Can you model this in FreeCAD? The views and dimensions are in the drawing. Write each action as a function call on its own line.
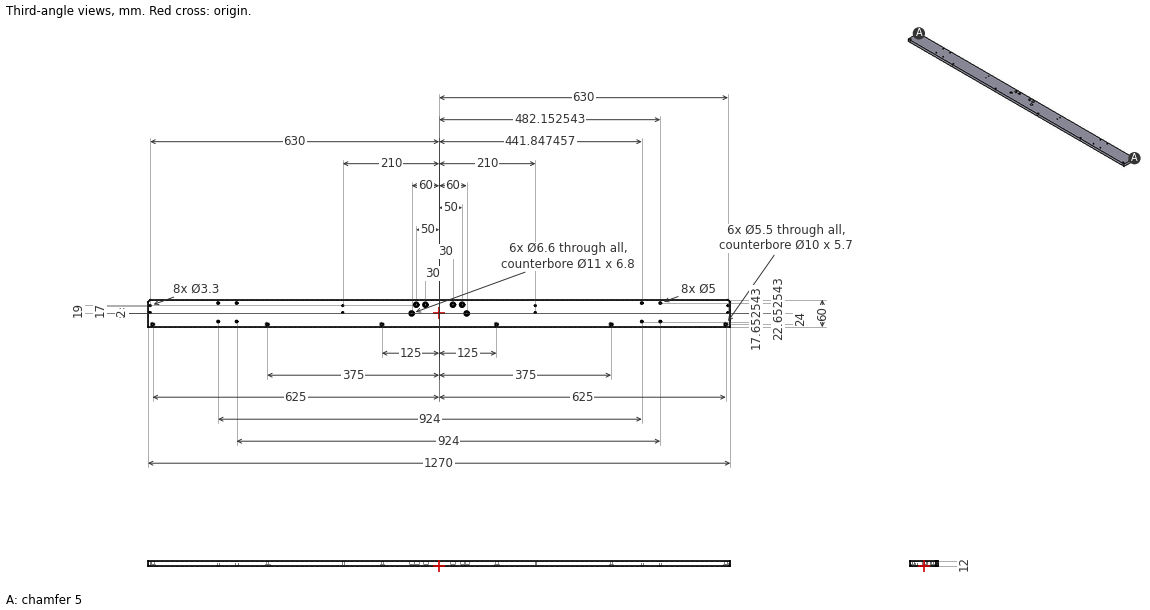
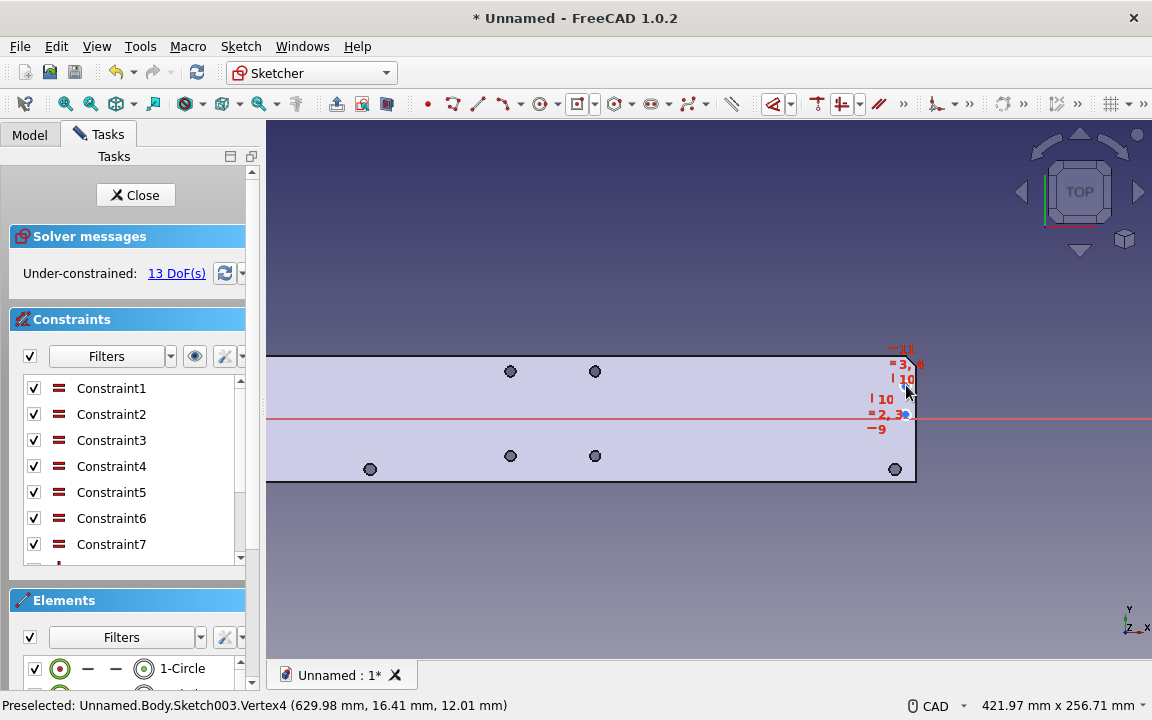
scroll(908, 387, down, 8)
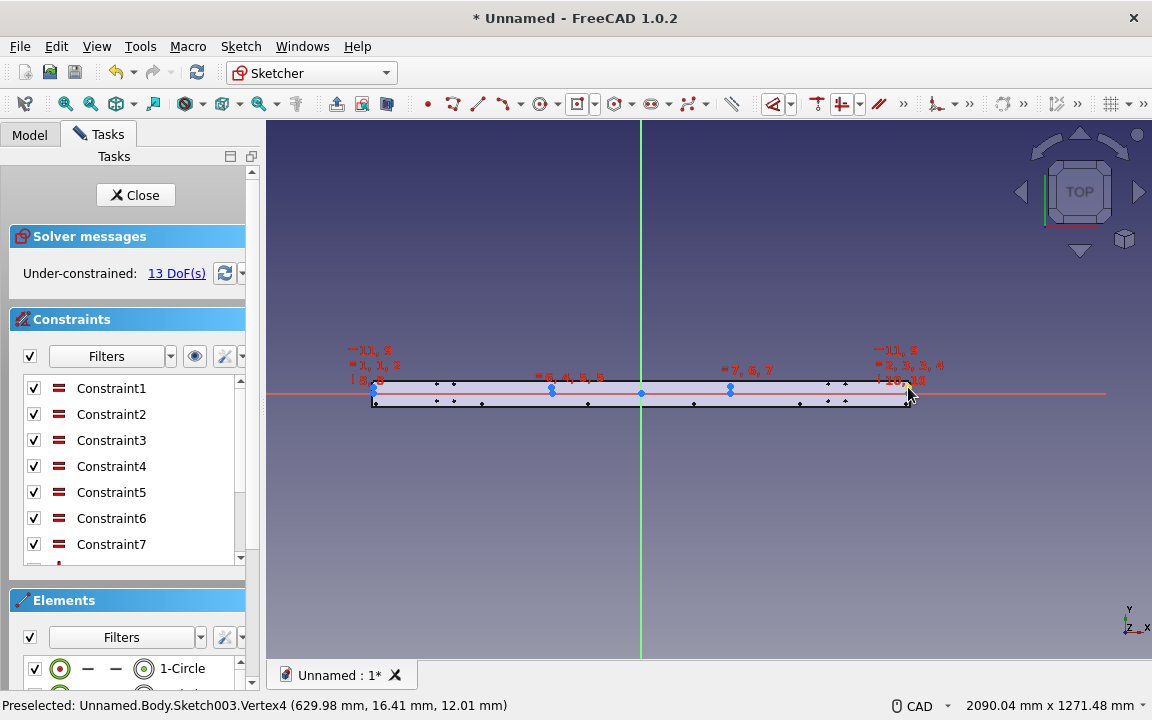
scroll(374, 387, up, 4)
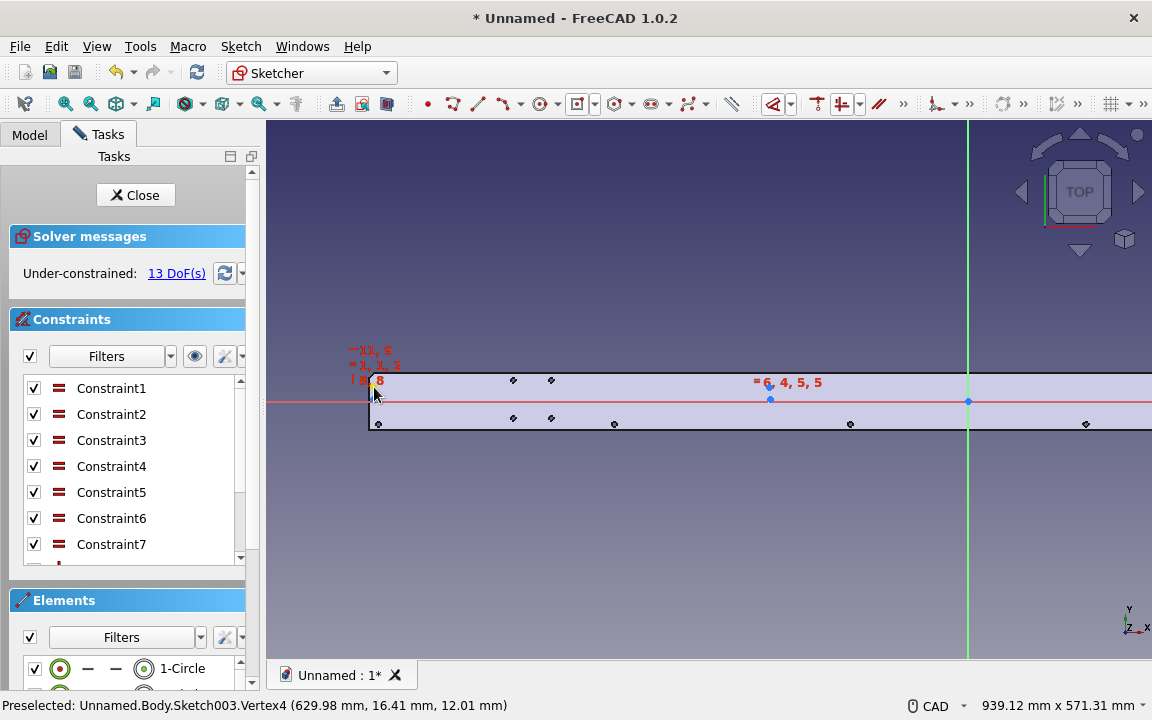
click(374, 387)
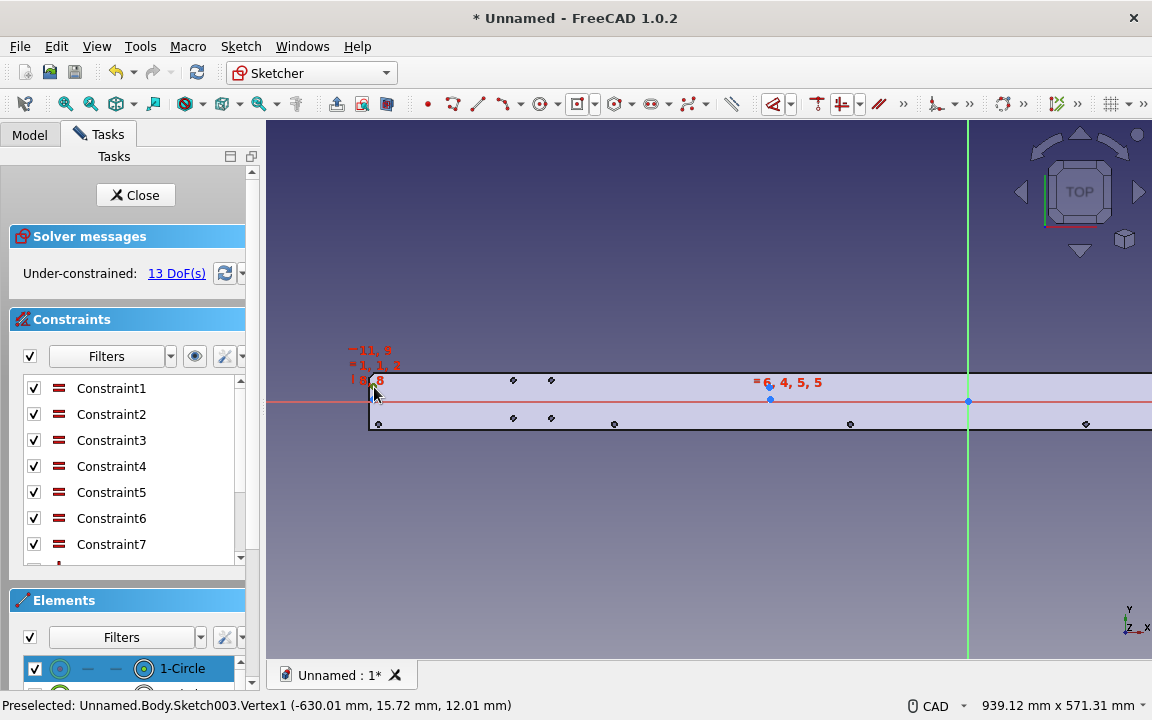
click(770, 387)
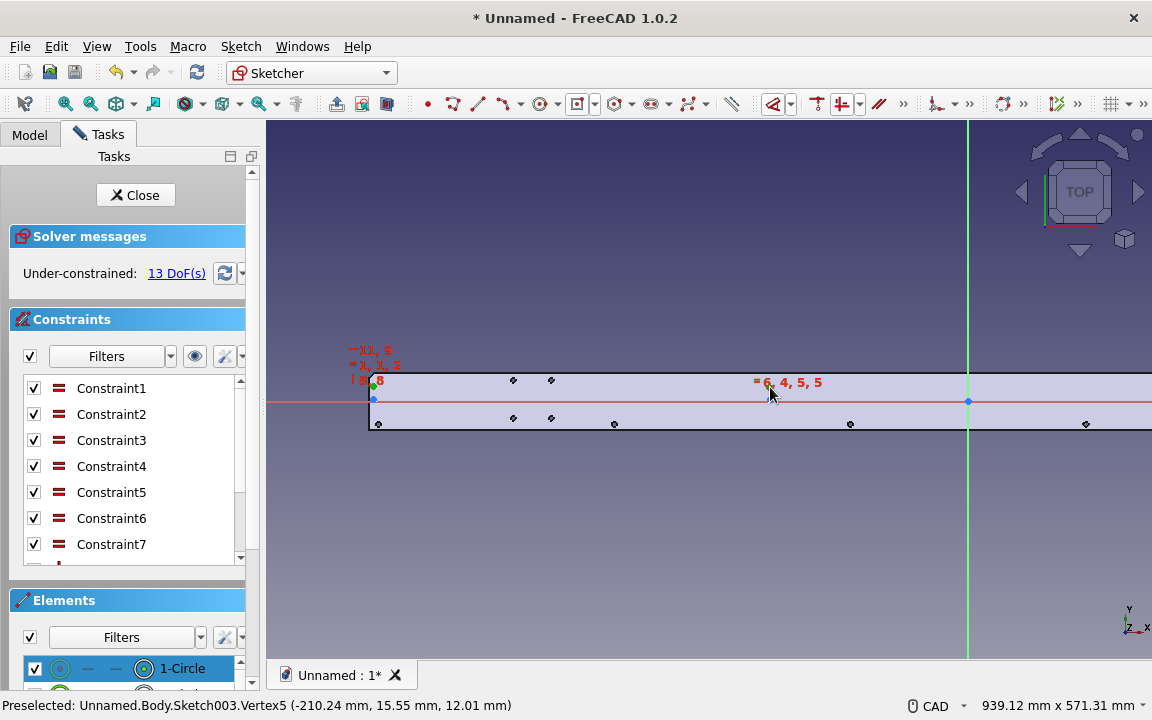
click(860, 104)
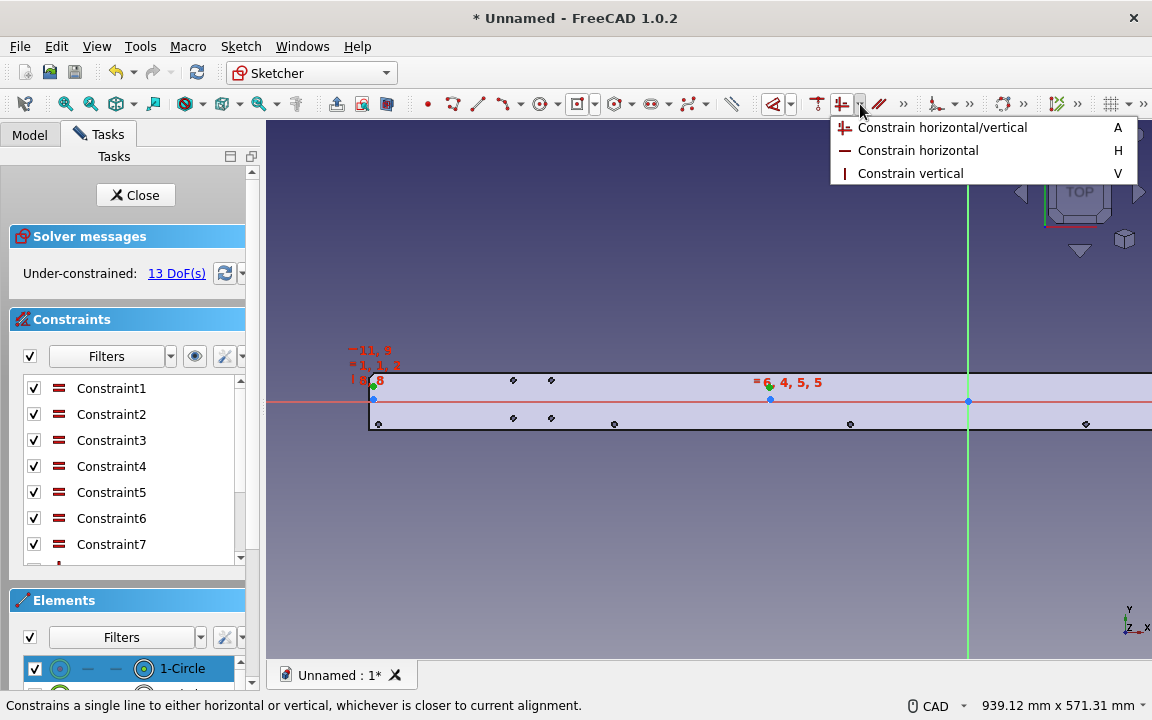
click(984, 150)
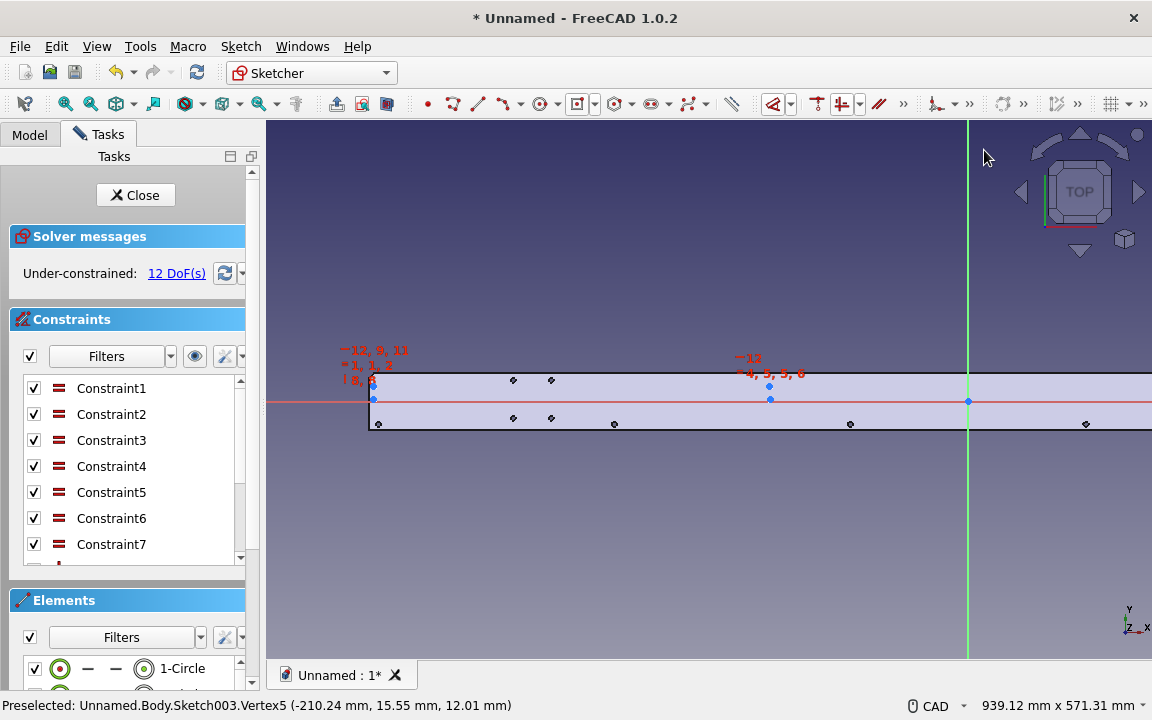
click(770, 387)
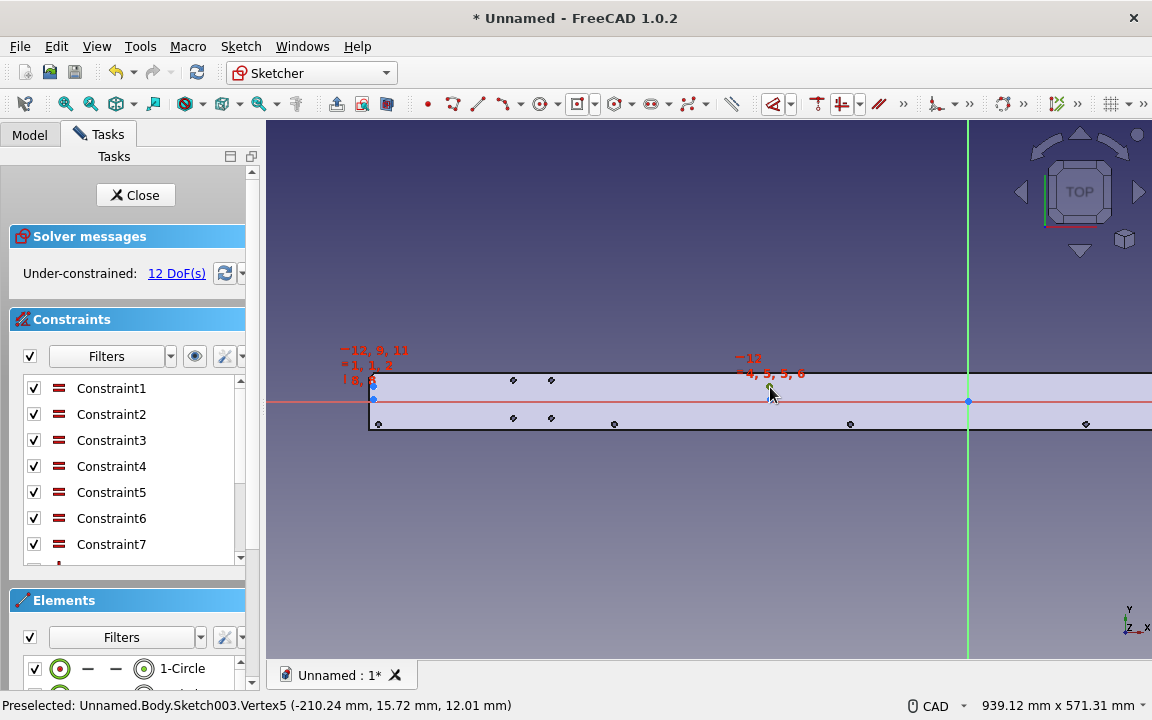
click(770, 400)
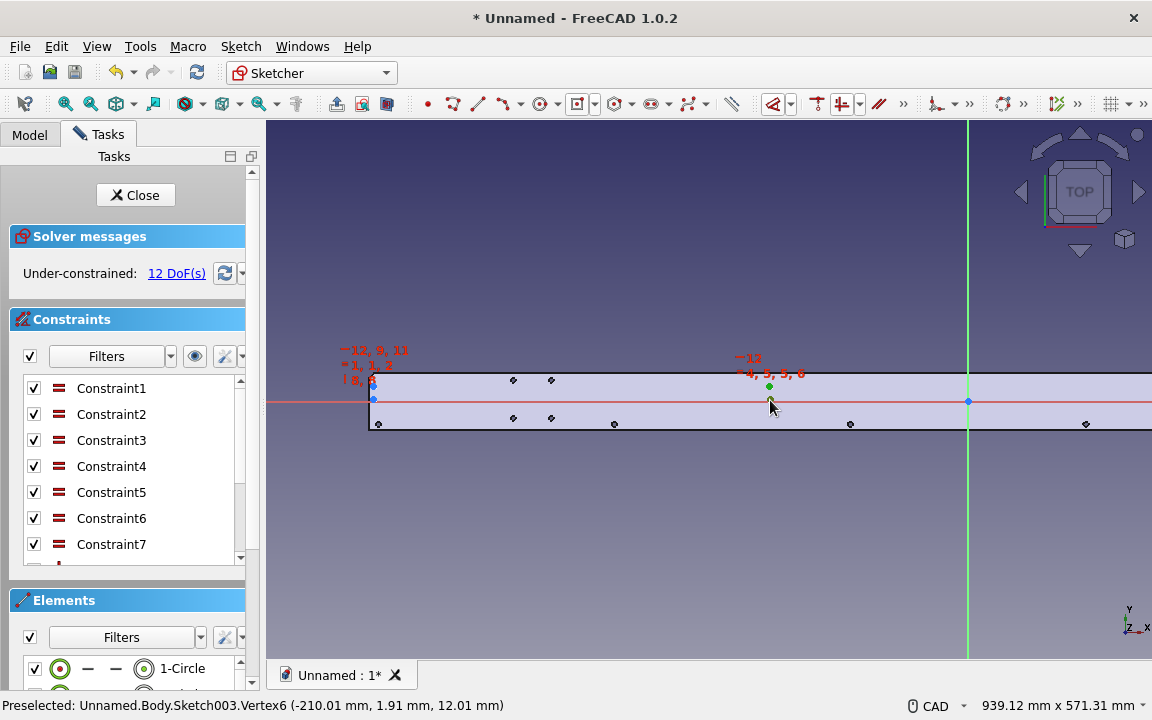
key(v)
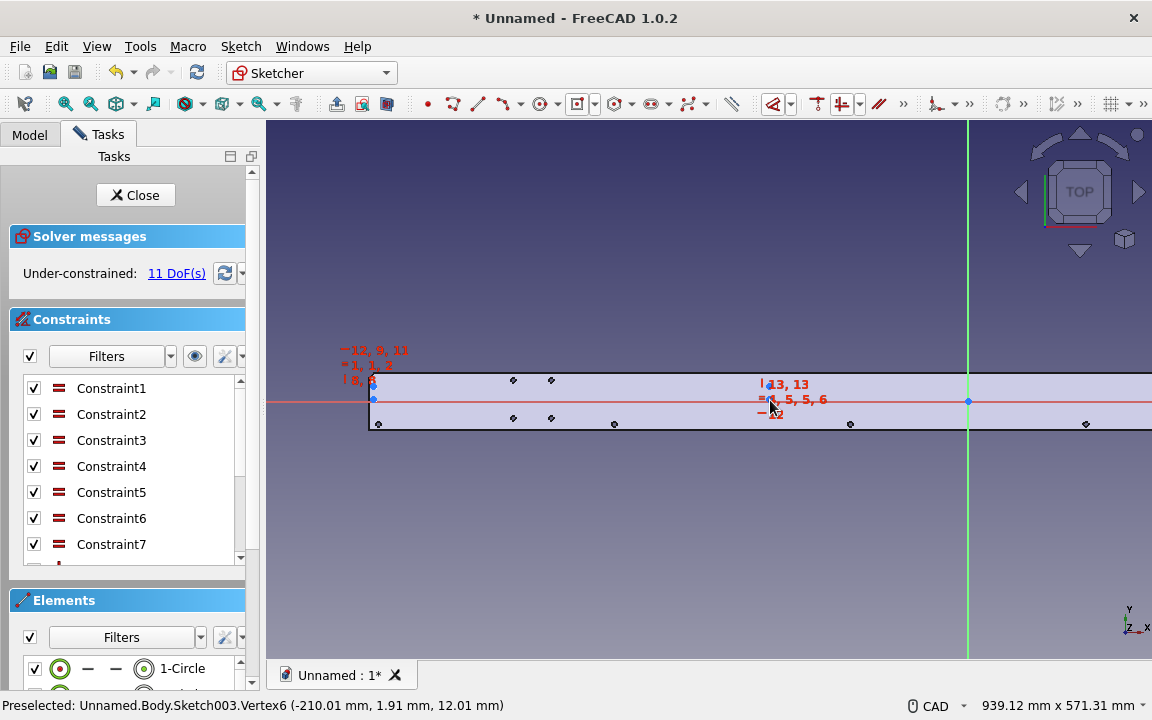
click(374, 400)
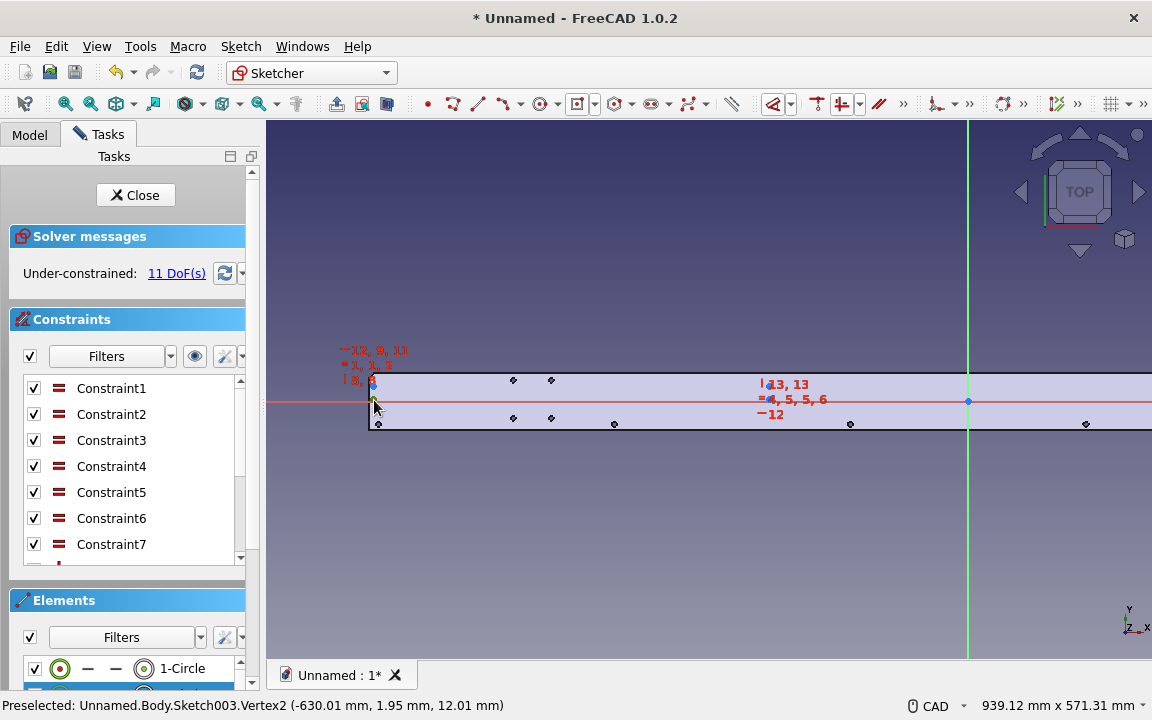
scroll(770, 400, up, 4)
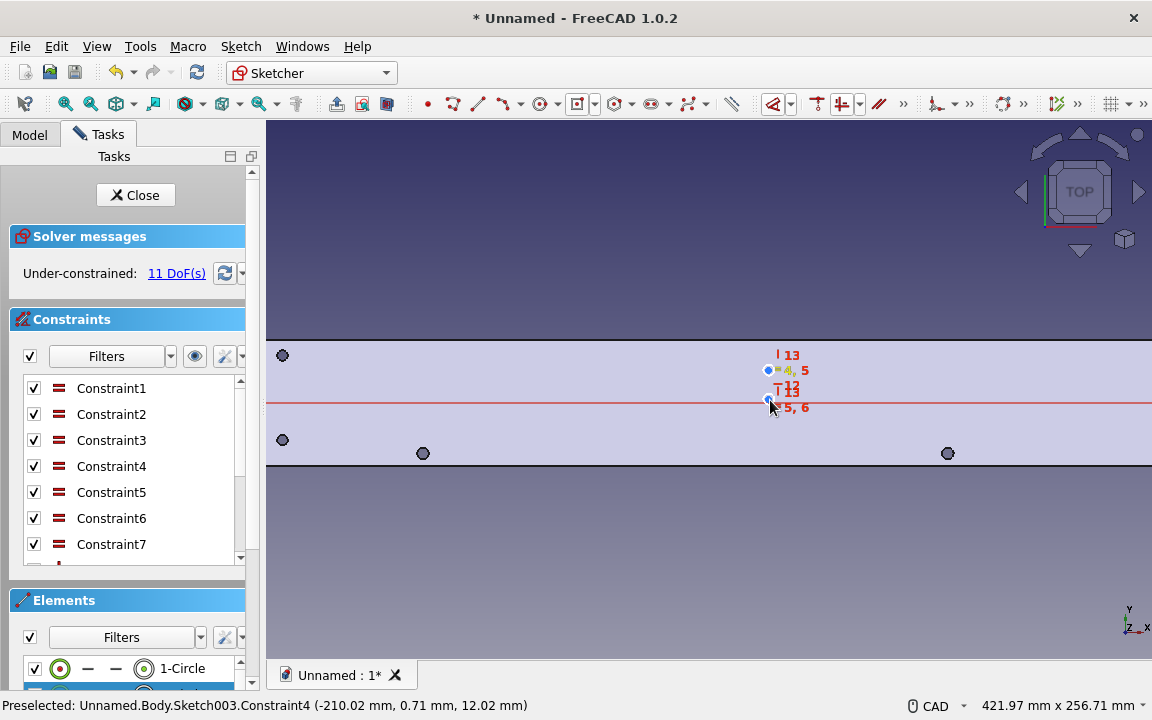
click(769, 399)